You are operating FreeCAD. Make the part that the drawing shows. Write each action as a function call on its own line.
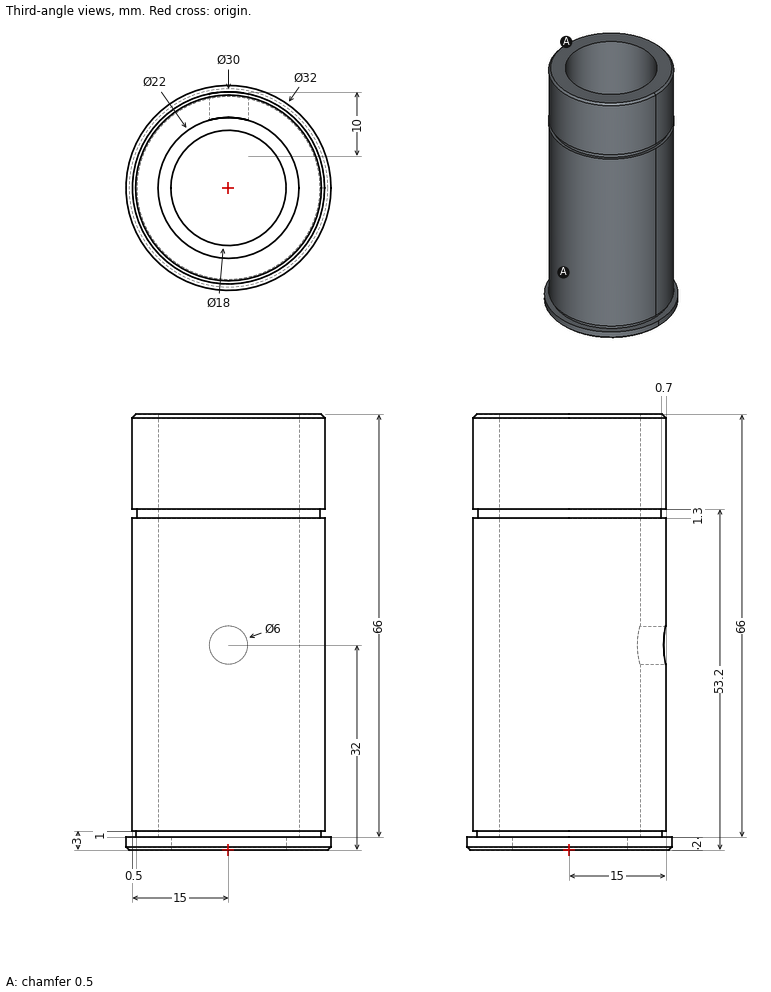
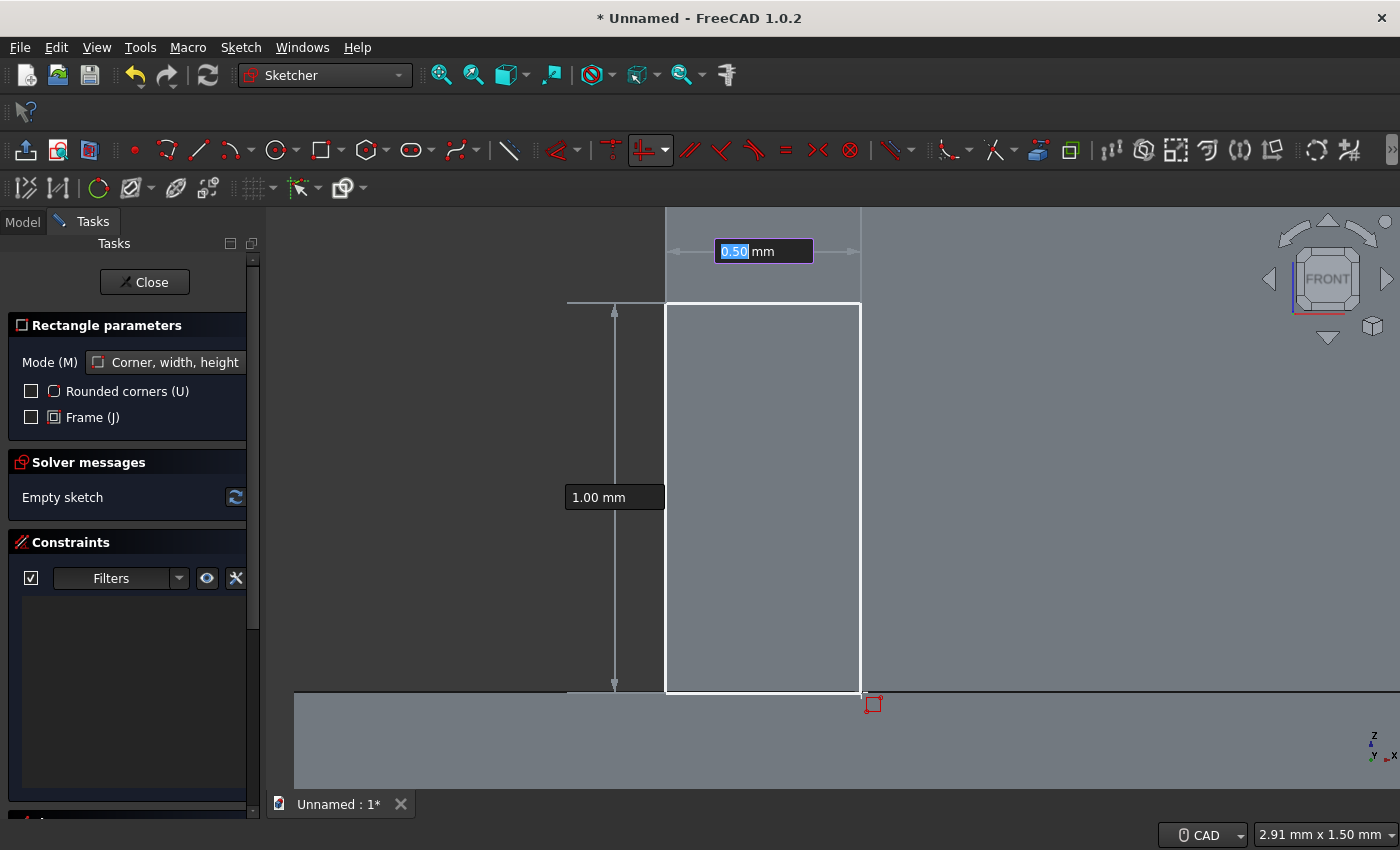
text(0.5)
key(Tab)
text(1)
key(Return)
key(Escape)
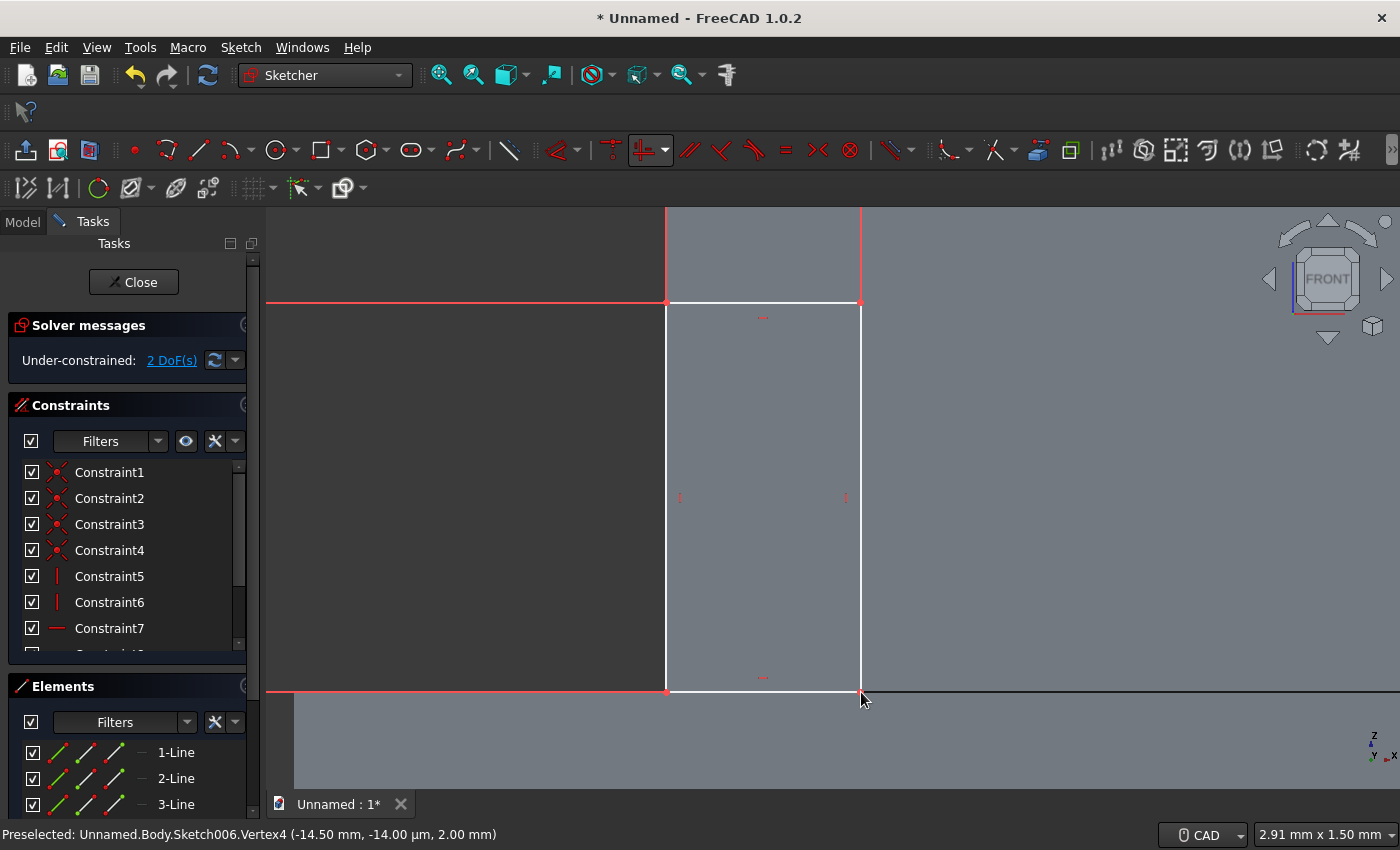
click(556, 150)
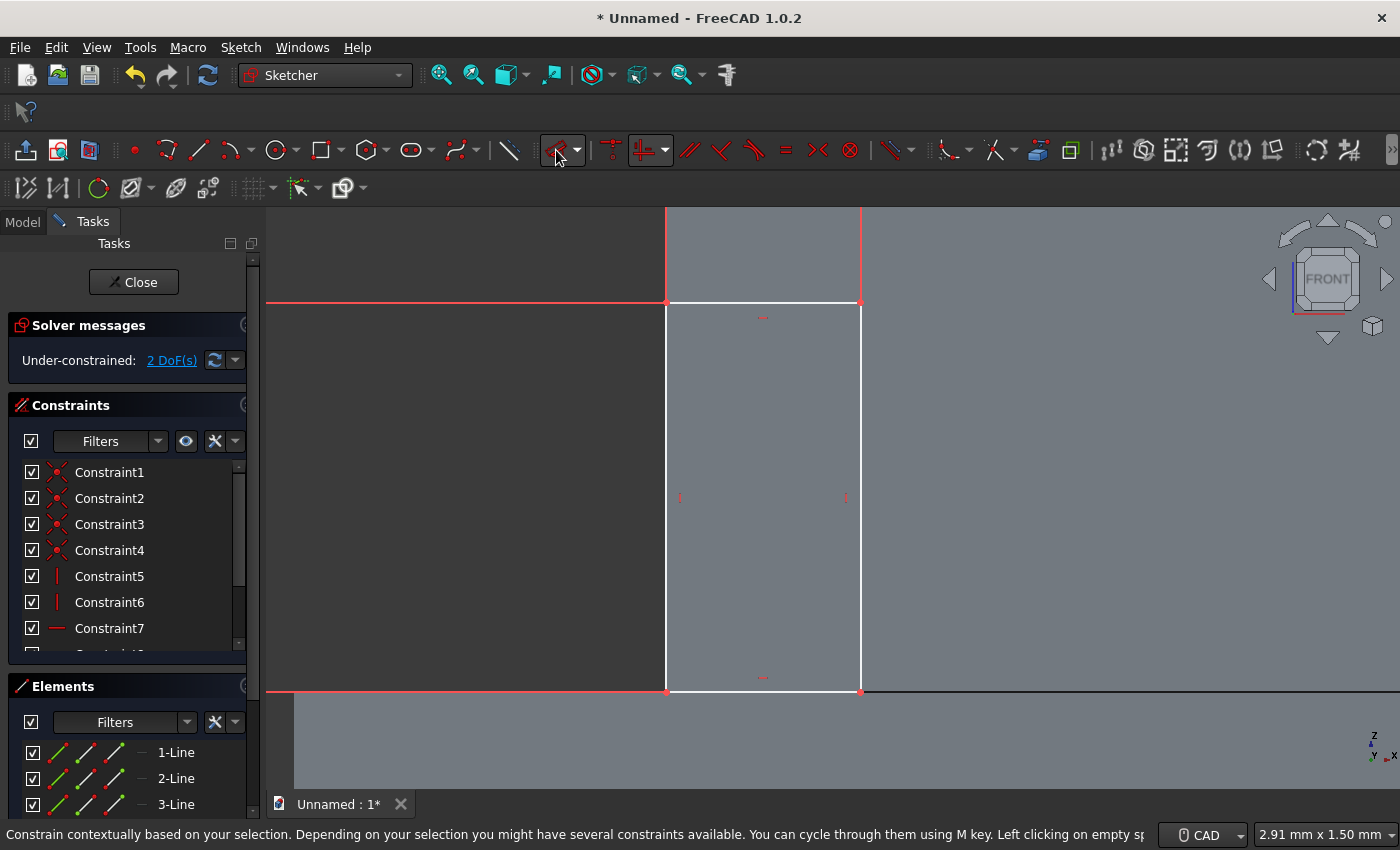
click(666, 303)
click(632, 532)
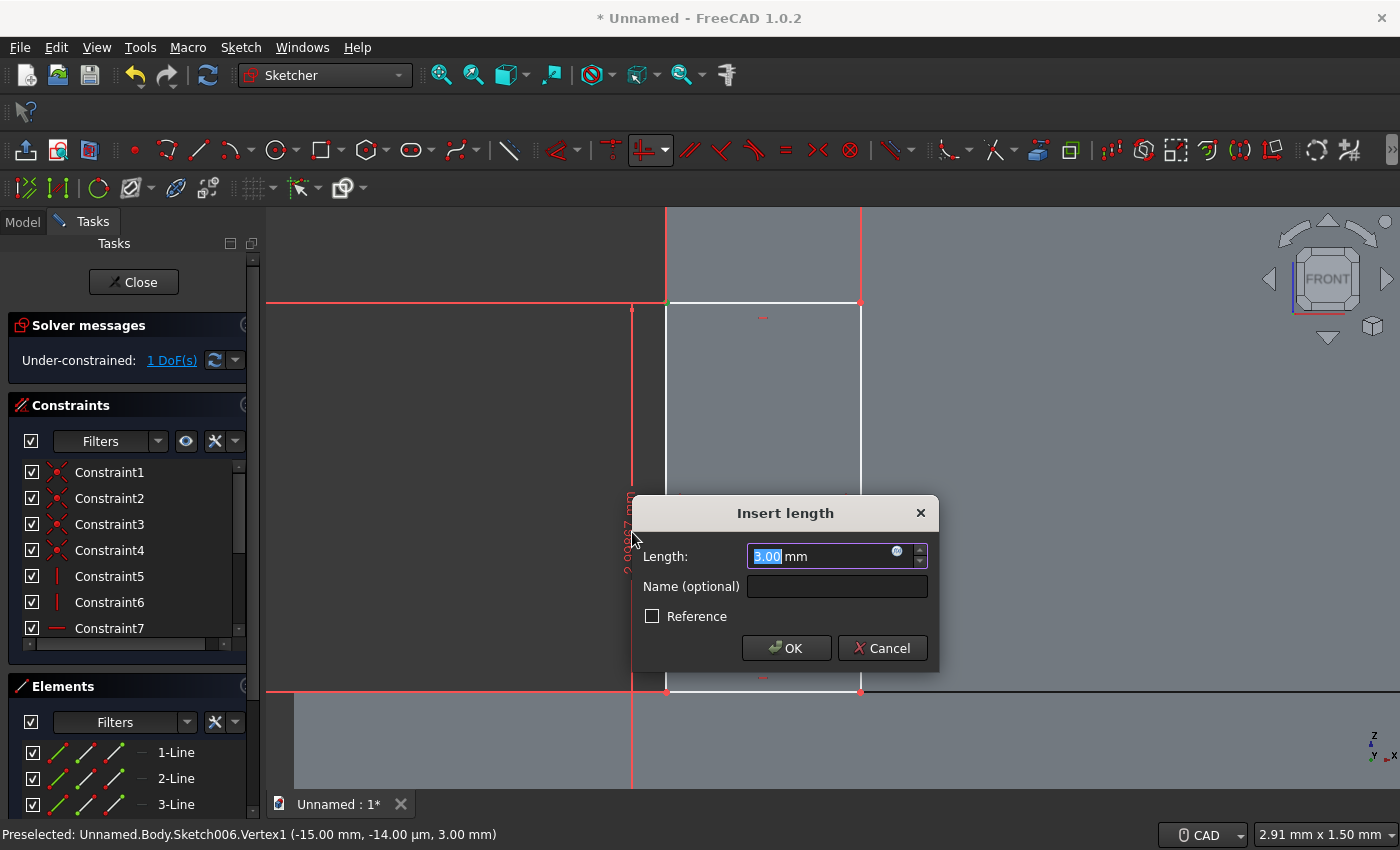
text(3)
key(Return)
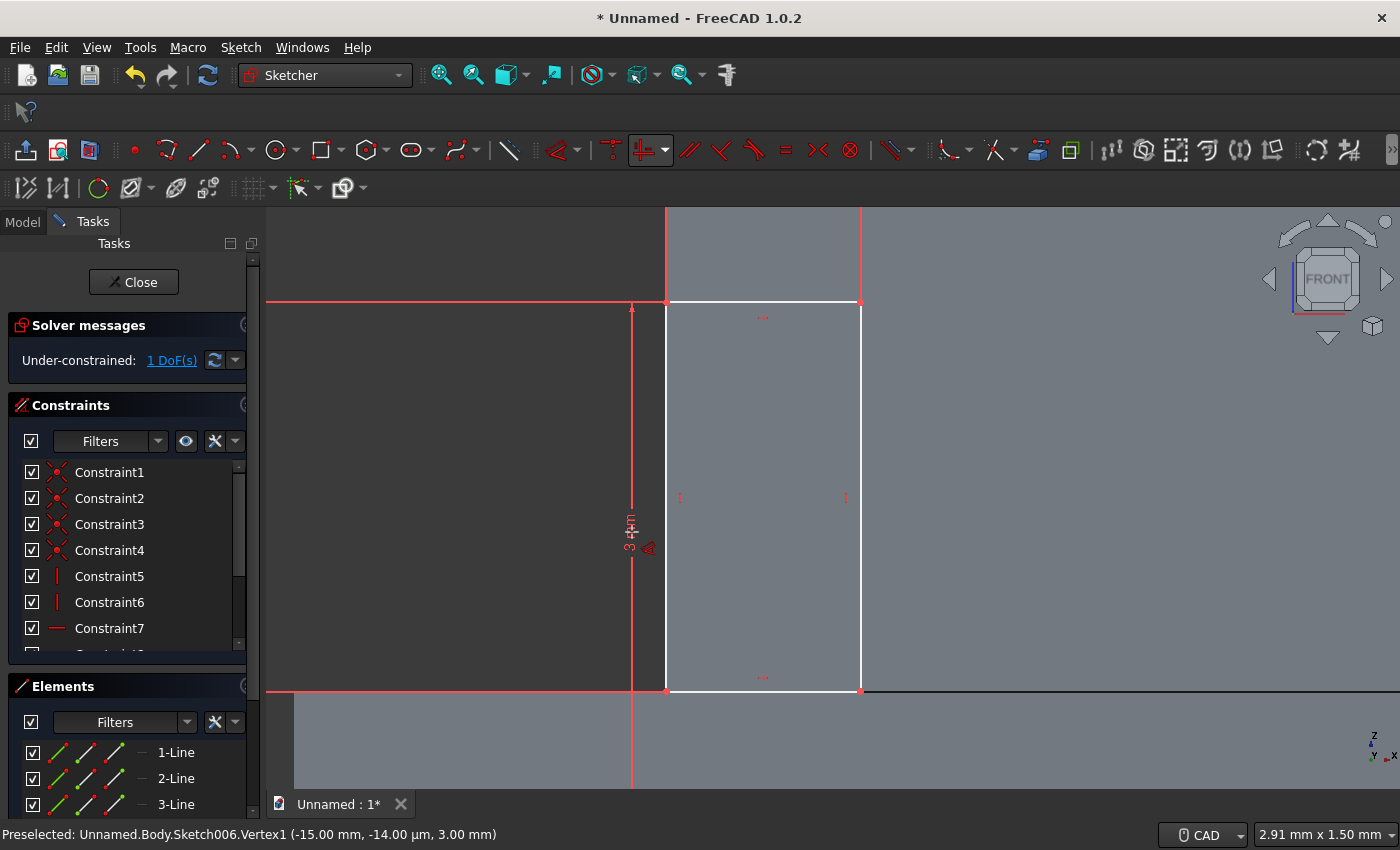
click(666, 302)
click(950, 268)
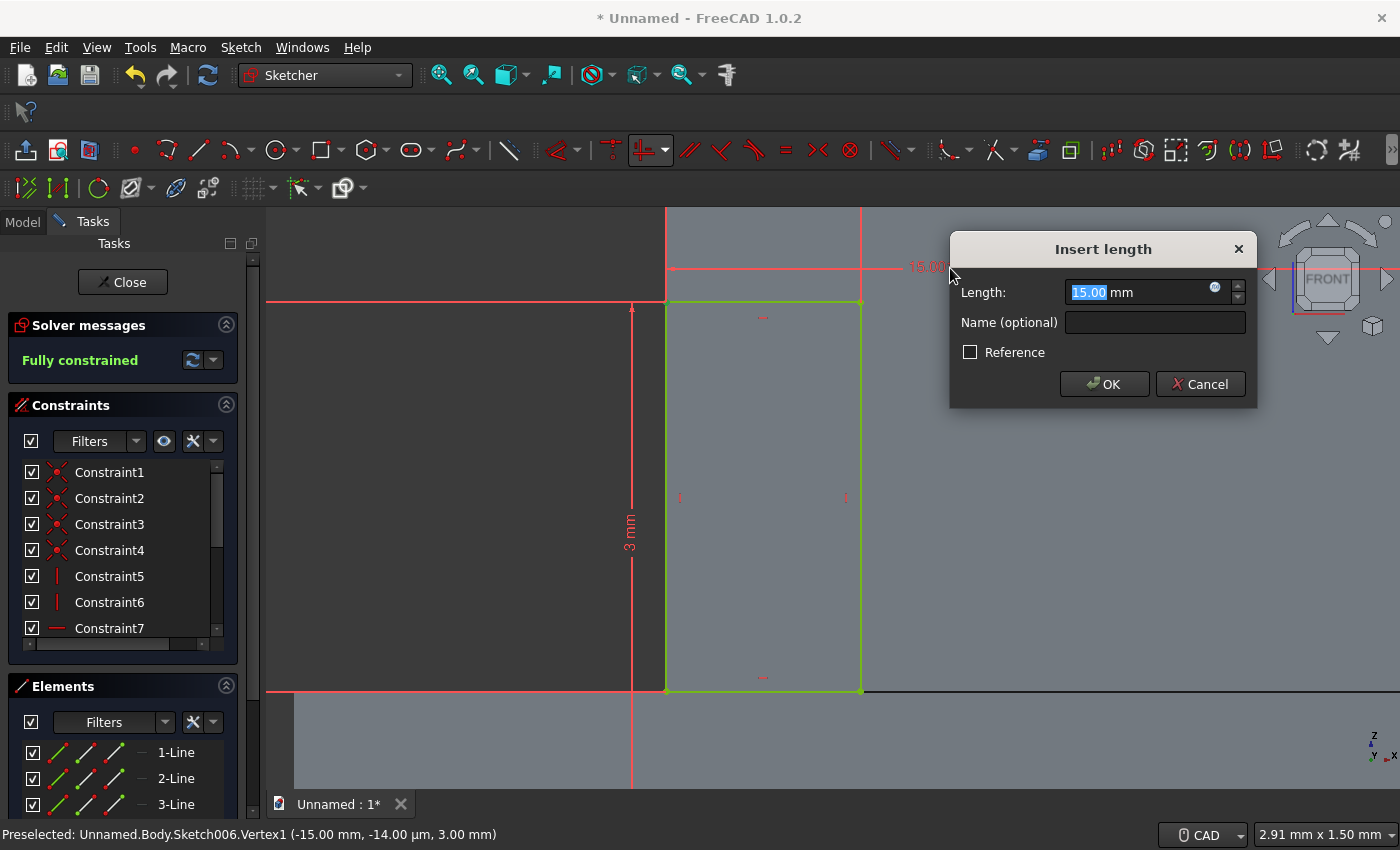
text(15)
key(Return)
key(Escape)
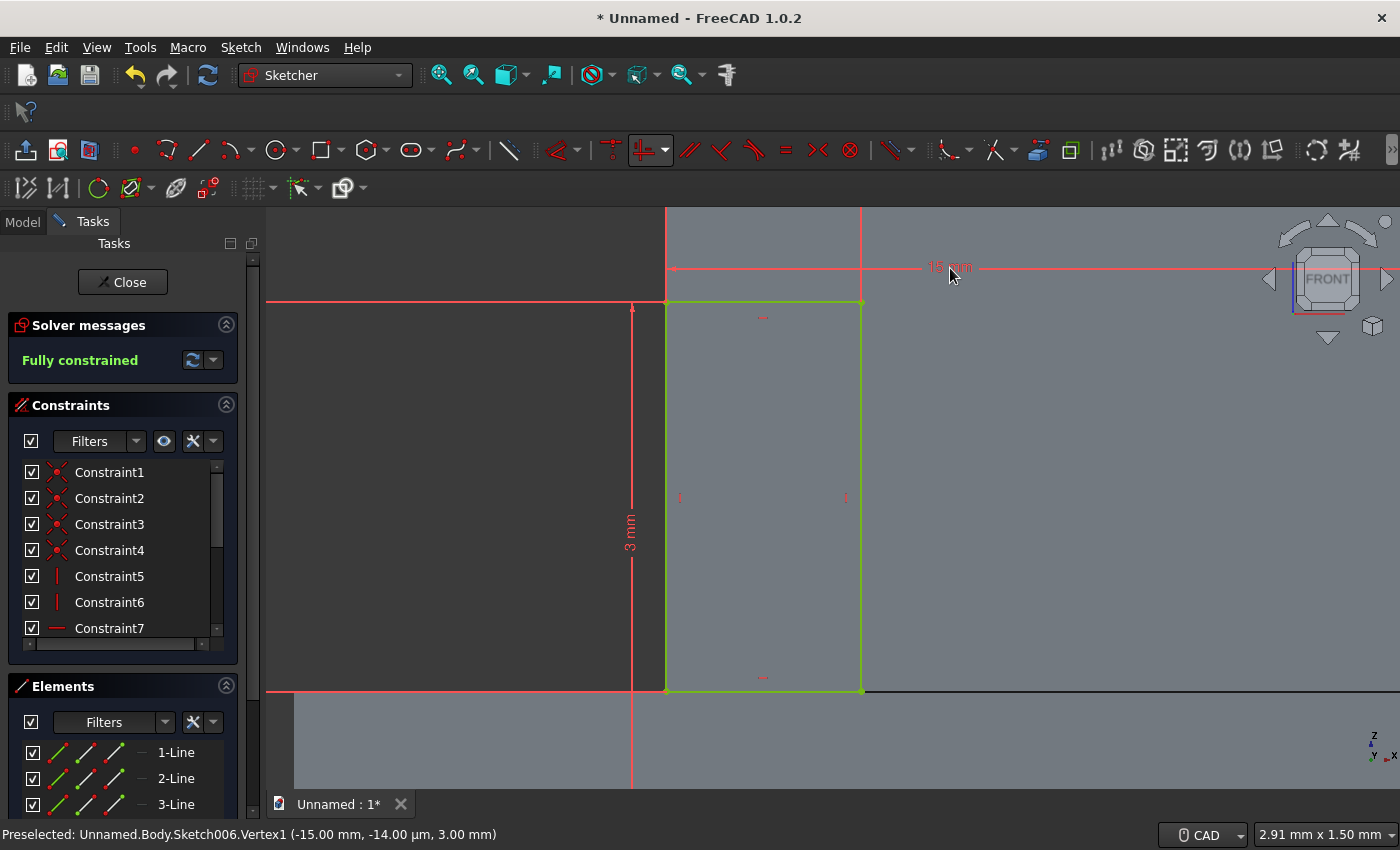
click(123, 282)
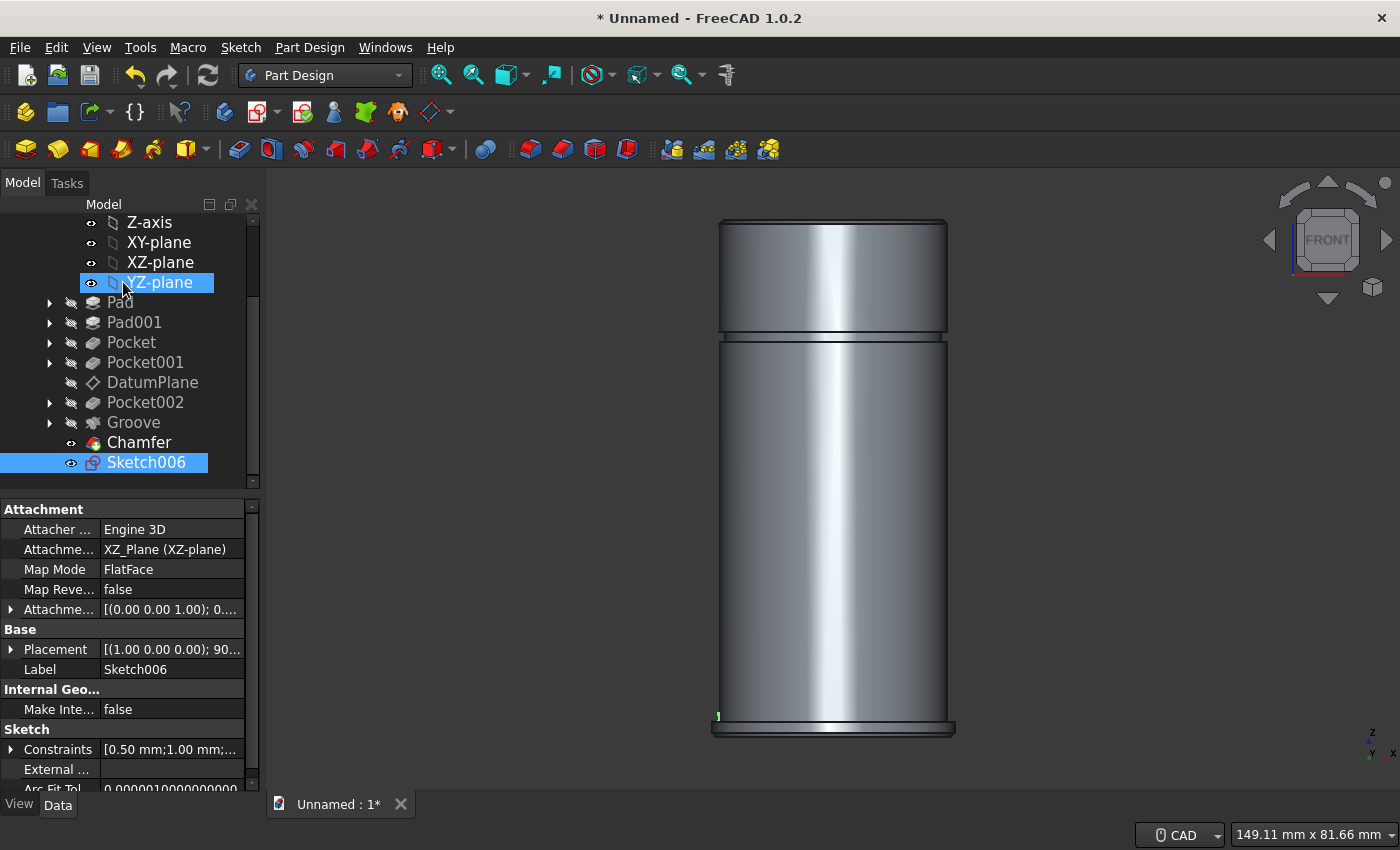
click(304, 150)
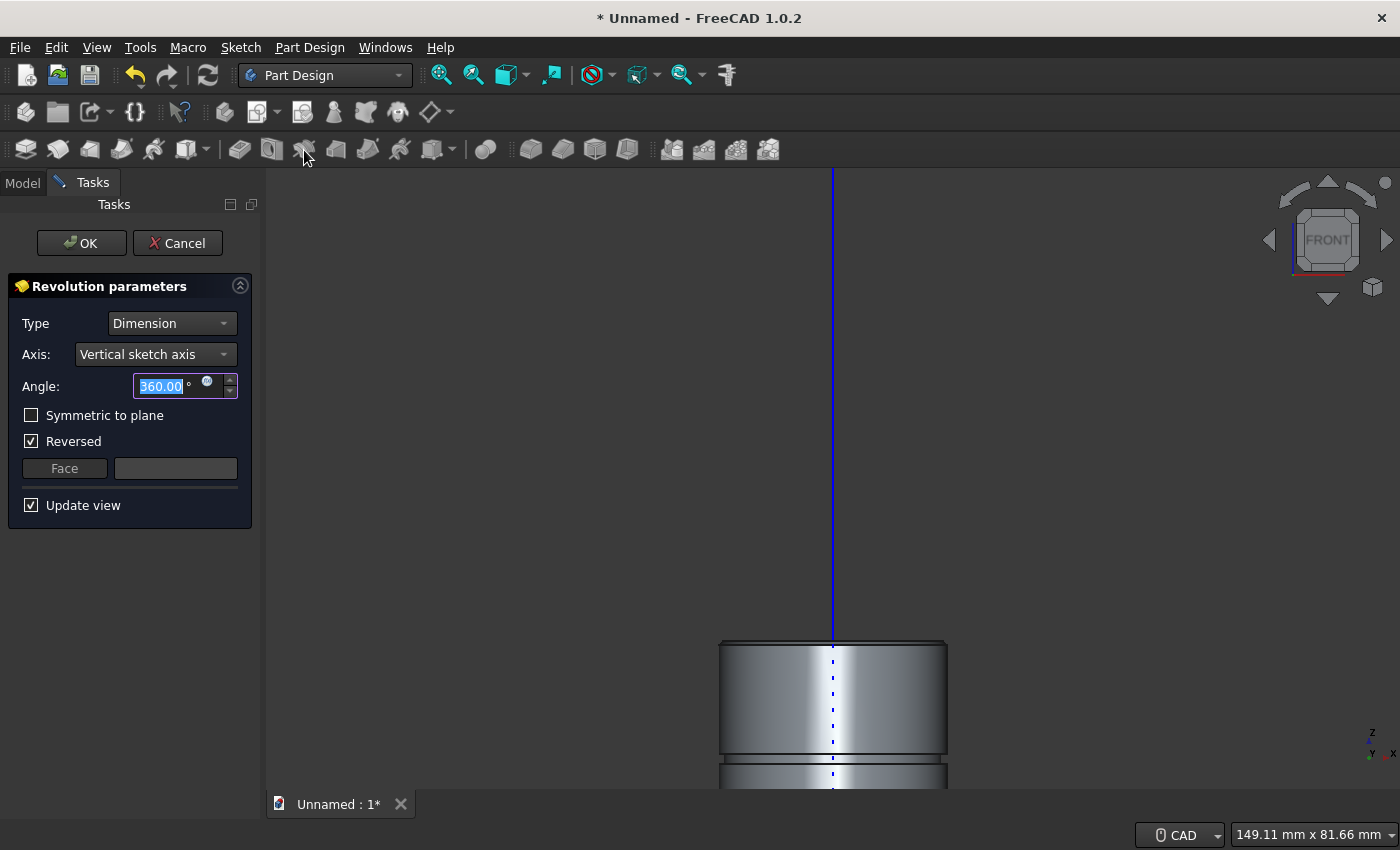
click(82, 243)